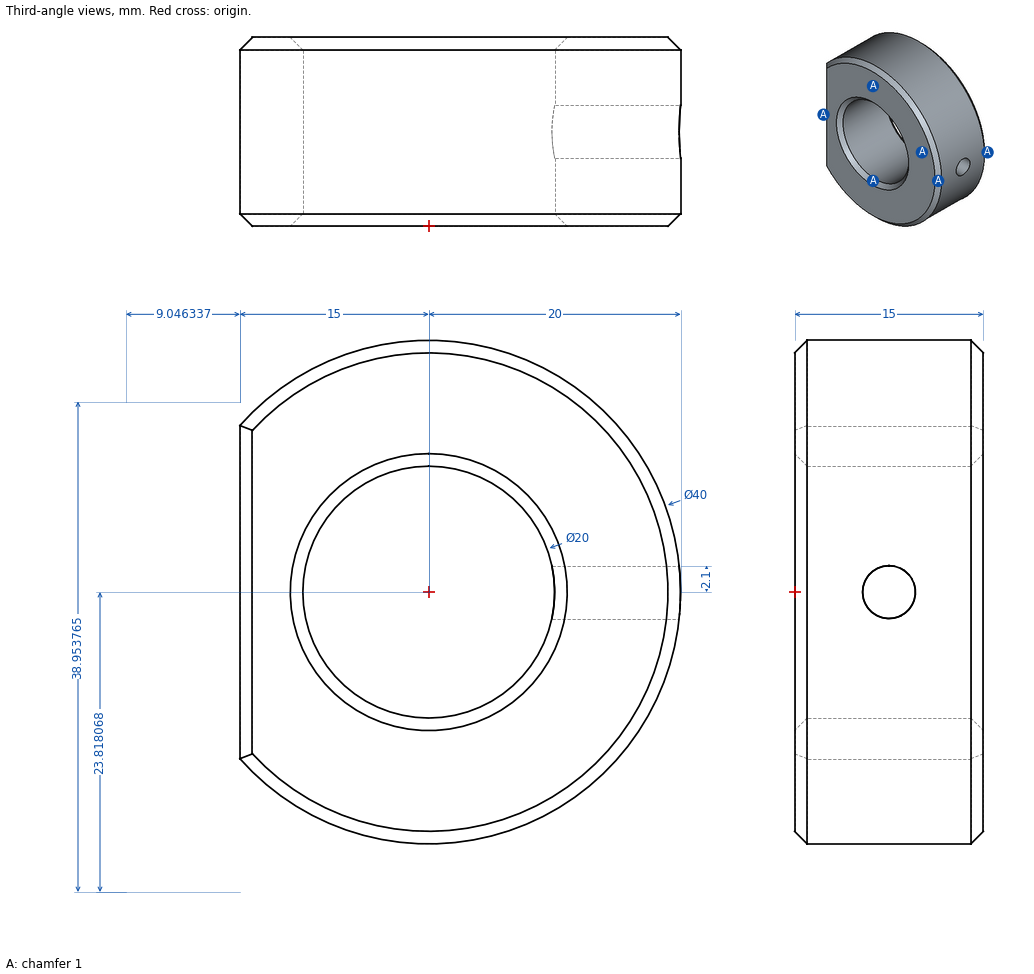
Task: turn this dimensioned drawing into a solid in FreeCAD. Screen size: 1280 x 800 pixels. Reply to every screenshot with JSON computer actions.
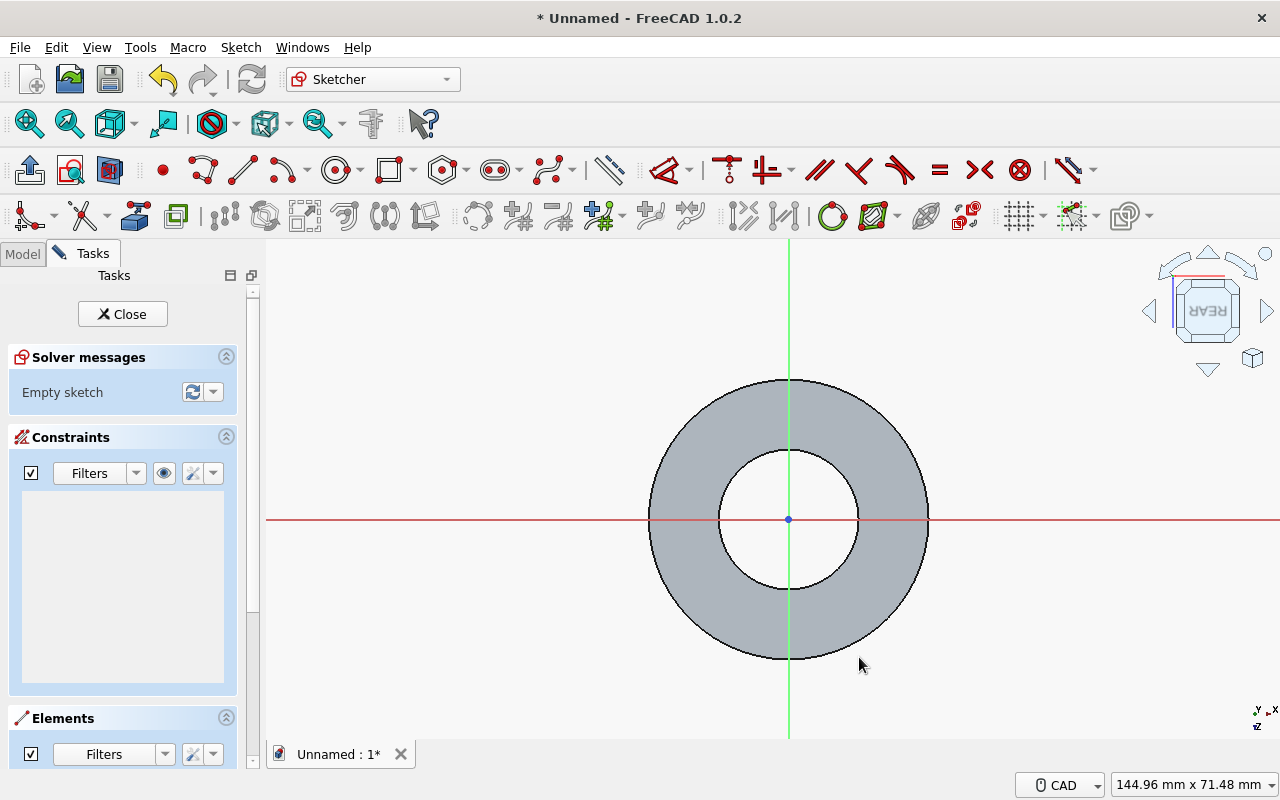
{"action": "left_click", "coordinate": [390, 170]}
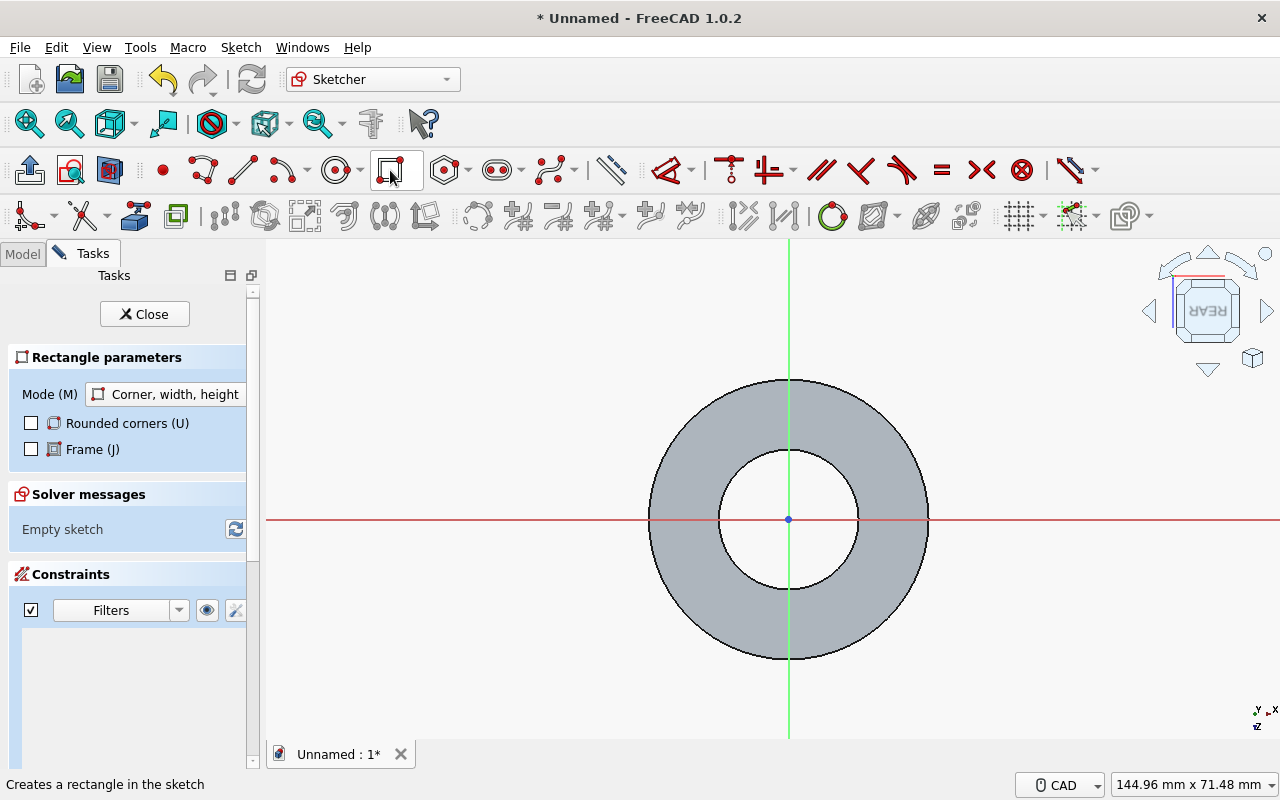
{"action": "left_click", "coordinate": [620, 353]}
{"action": "mouse_move", "coordinate": [684, 625]}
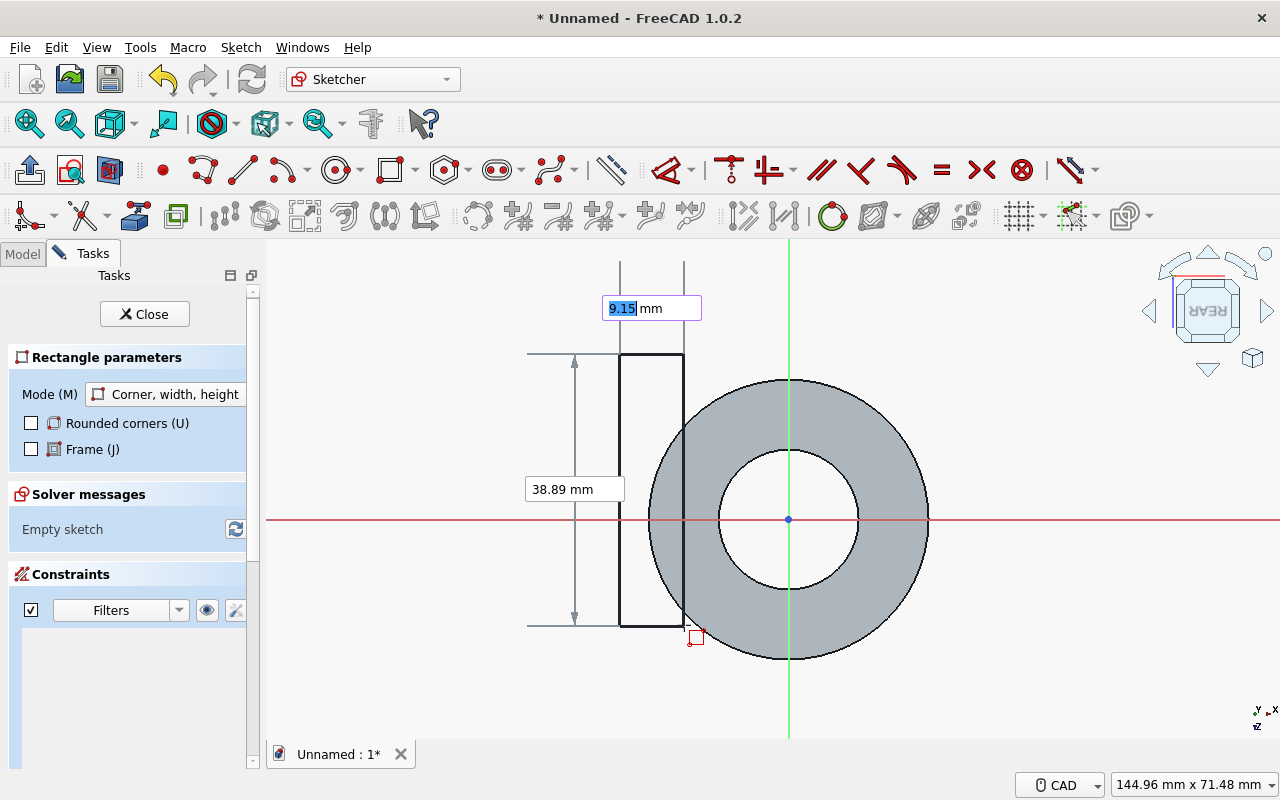
{"action": "type", "text": "9.046337"}
{"action": "key", "text": "Tab"}
{"action": "type", "text": "38.953765"}
{"action": "key", "text": "Return"}
{"action": "key", "text": "Escape"}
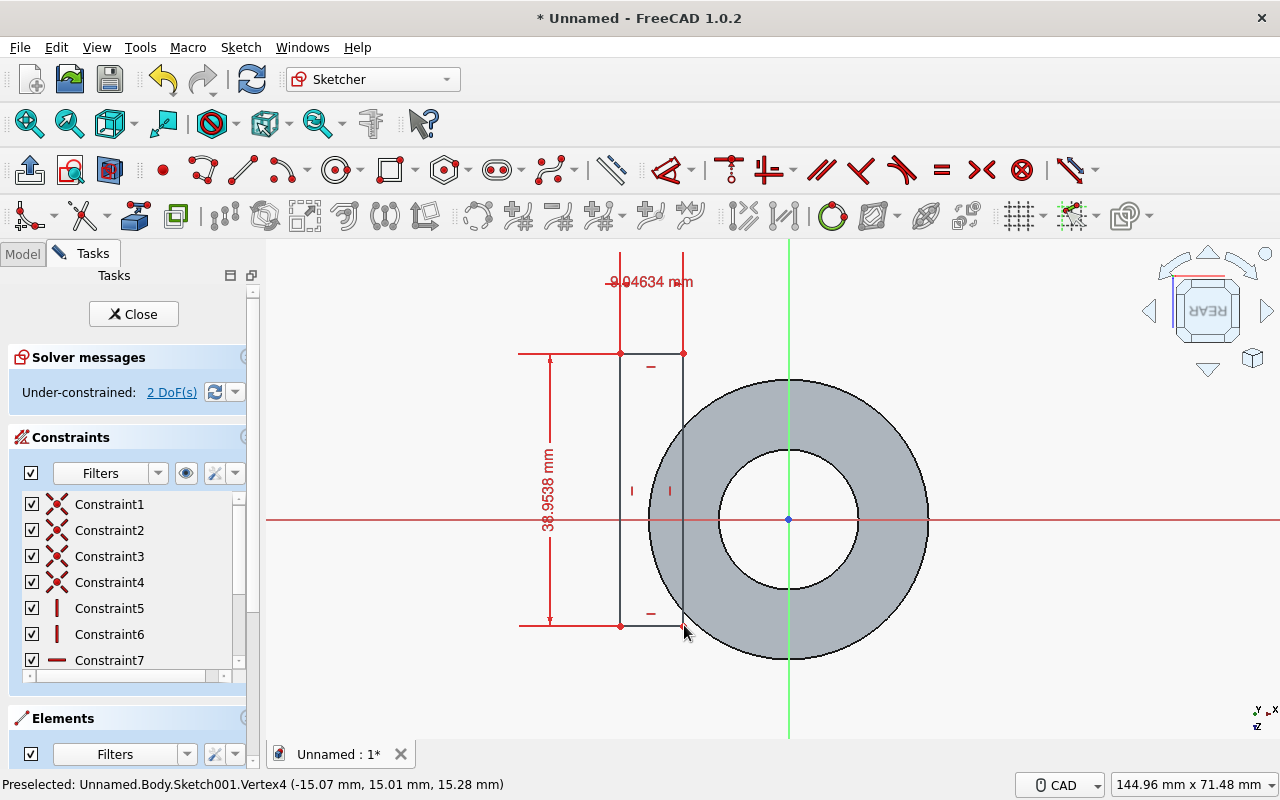
{"action": "left_click", "coordinate": [666, 170]}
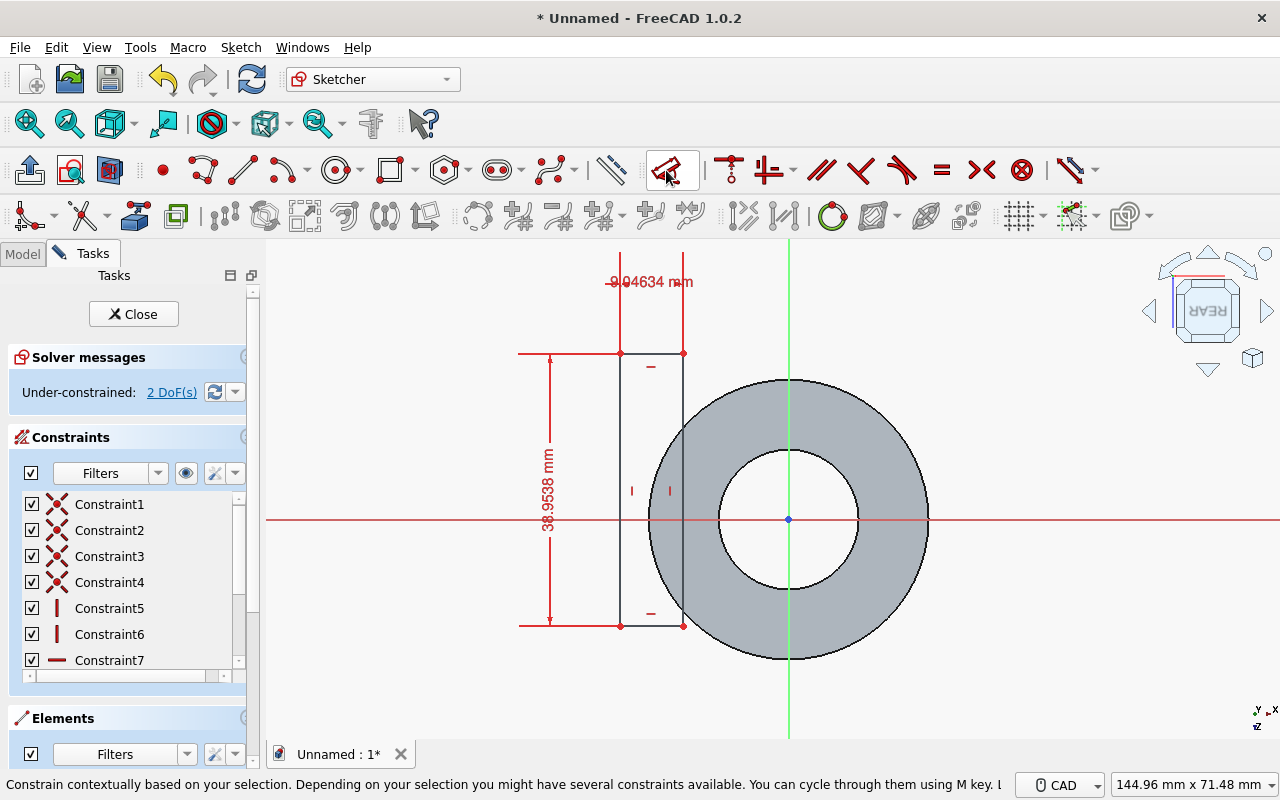
{"action": "left_click", "coordinate": [683, 626]}
{"action": "left_click", "coordinate": [736, 660]}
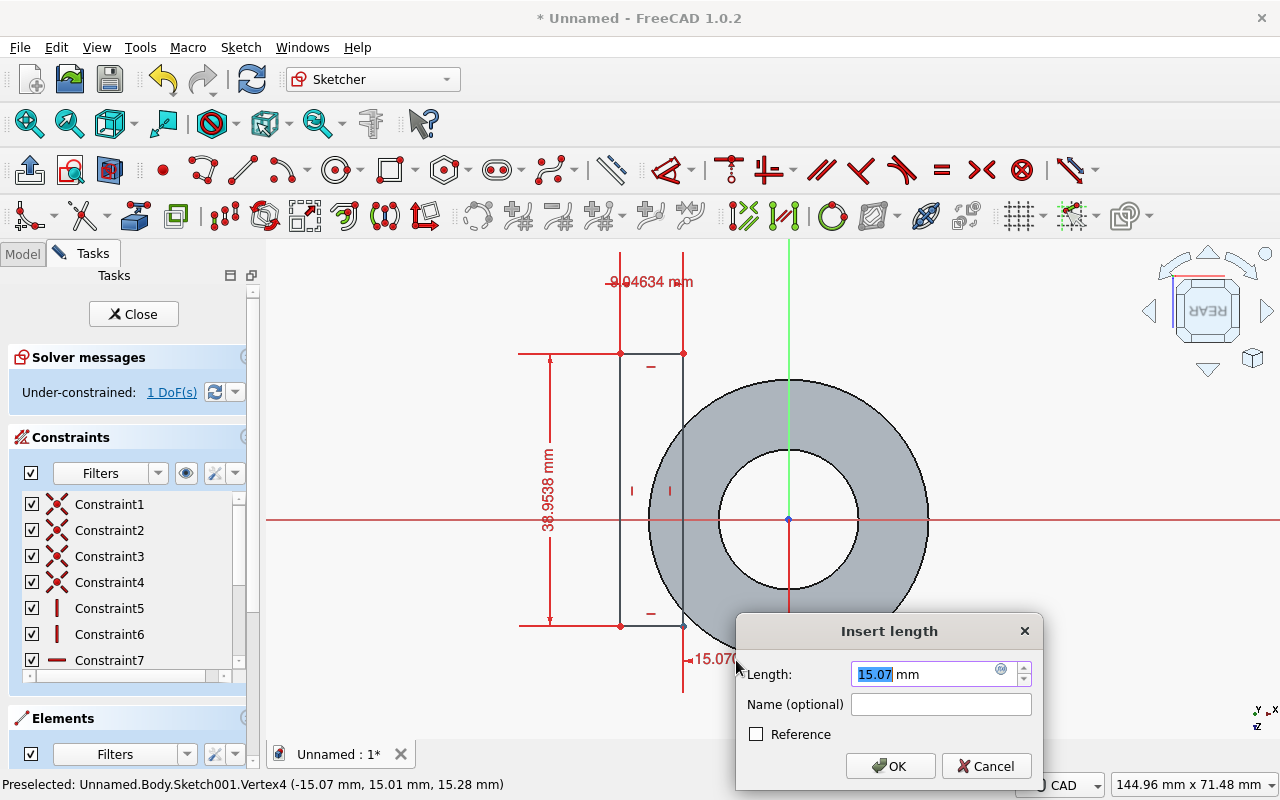
{"action": "type", "text": "15"}
{"action": "key", "text": "Return"}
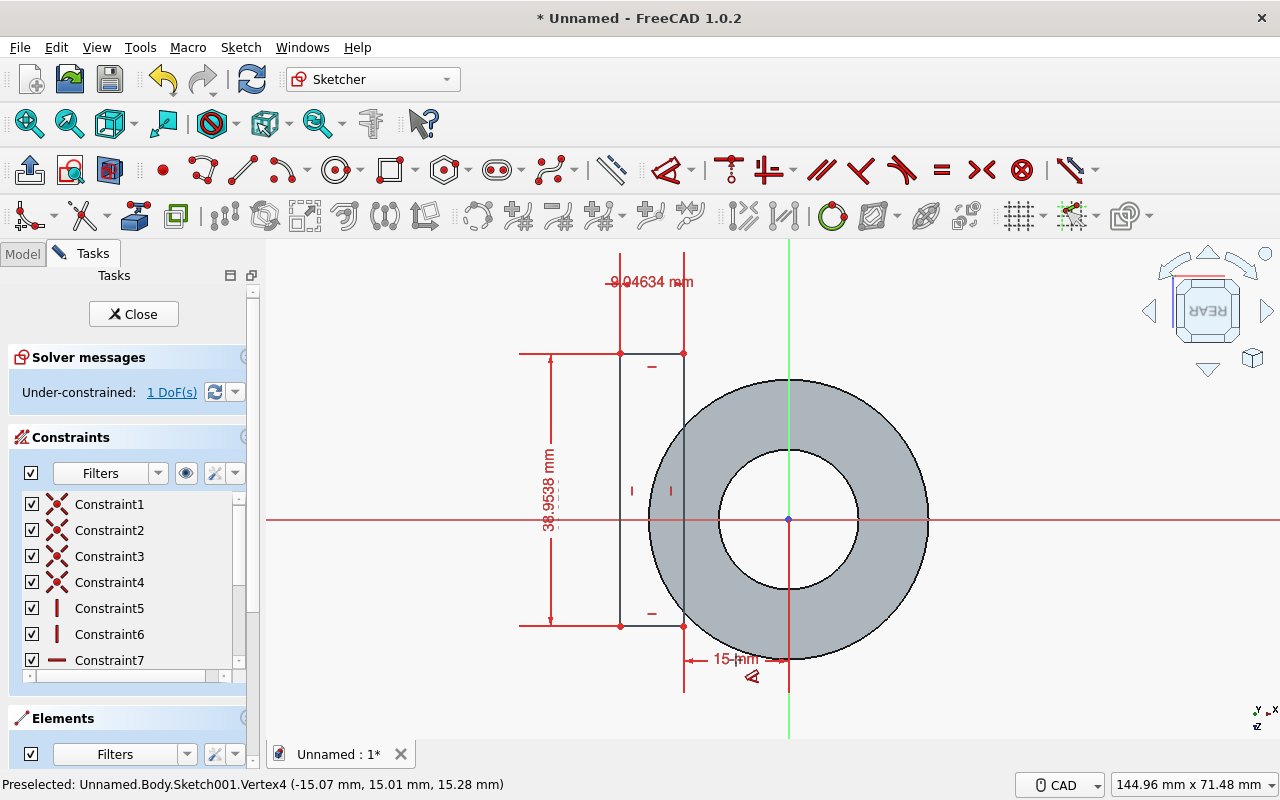
{"action": "left_click", "coordinate": [620, 354]}
{"action": "left_click", "coordinate": [586, 437]}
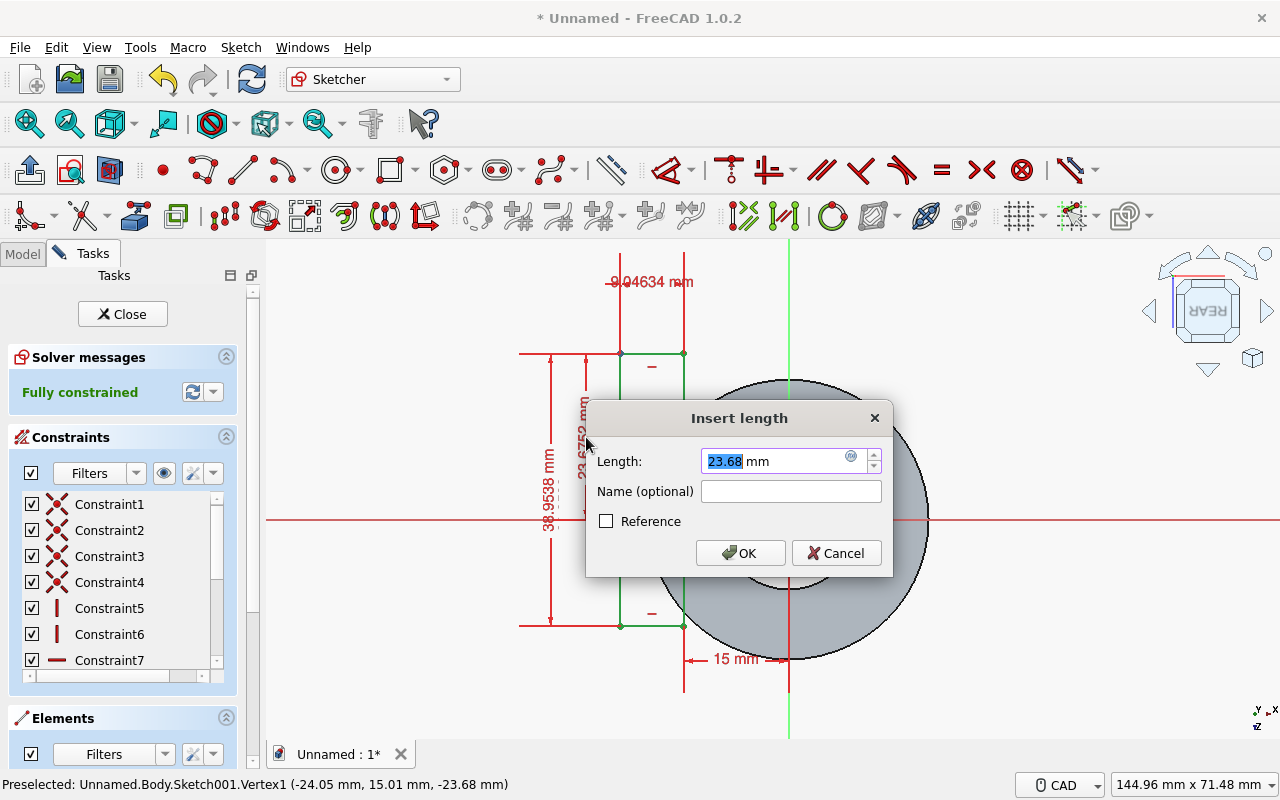
{"action": "type", "text": "23.818068"}
{"action": "key", "text": "Return"}
{"action": "key", "text": "Escape"}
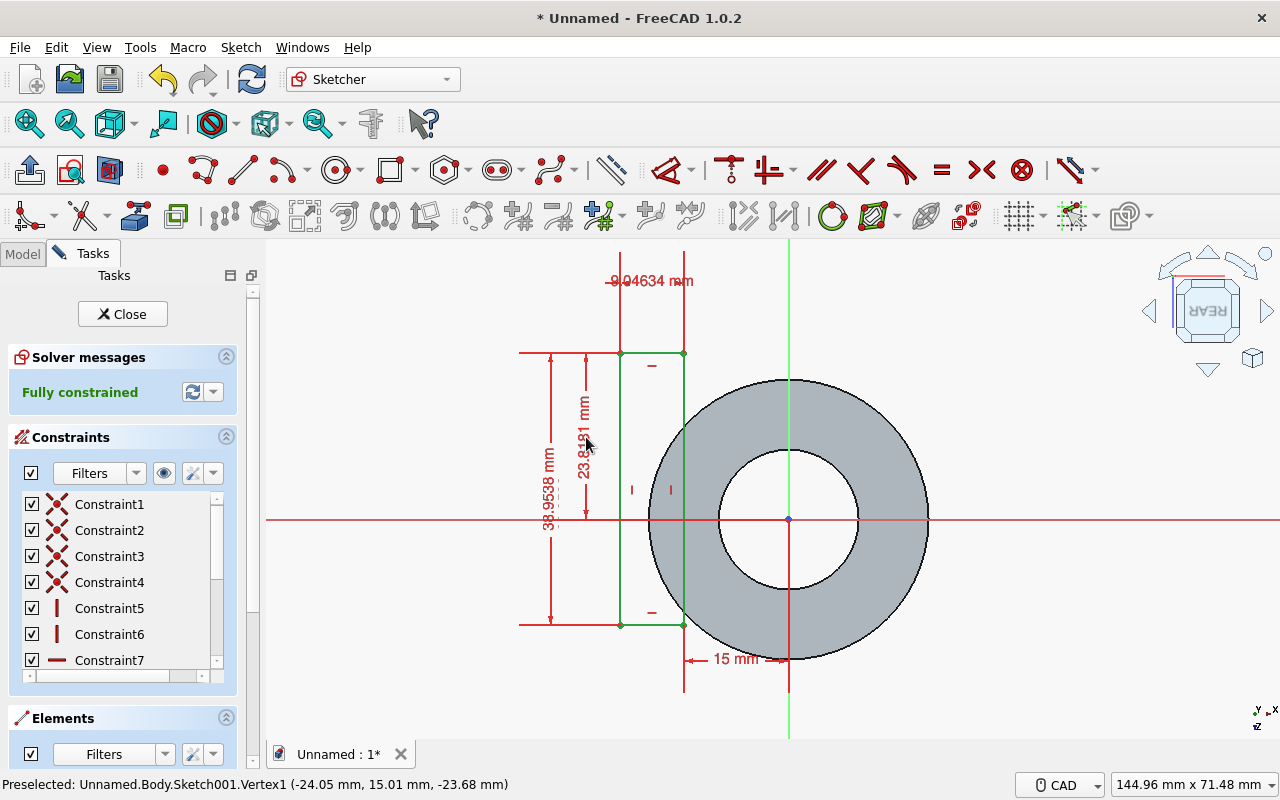
{"action": "left_click", "coordinate": [123, 314]}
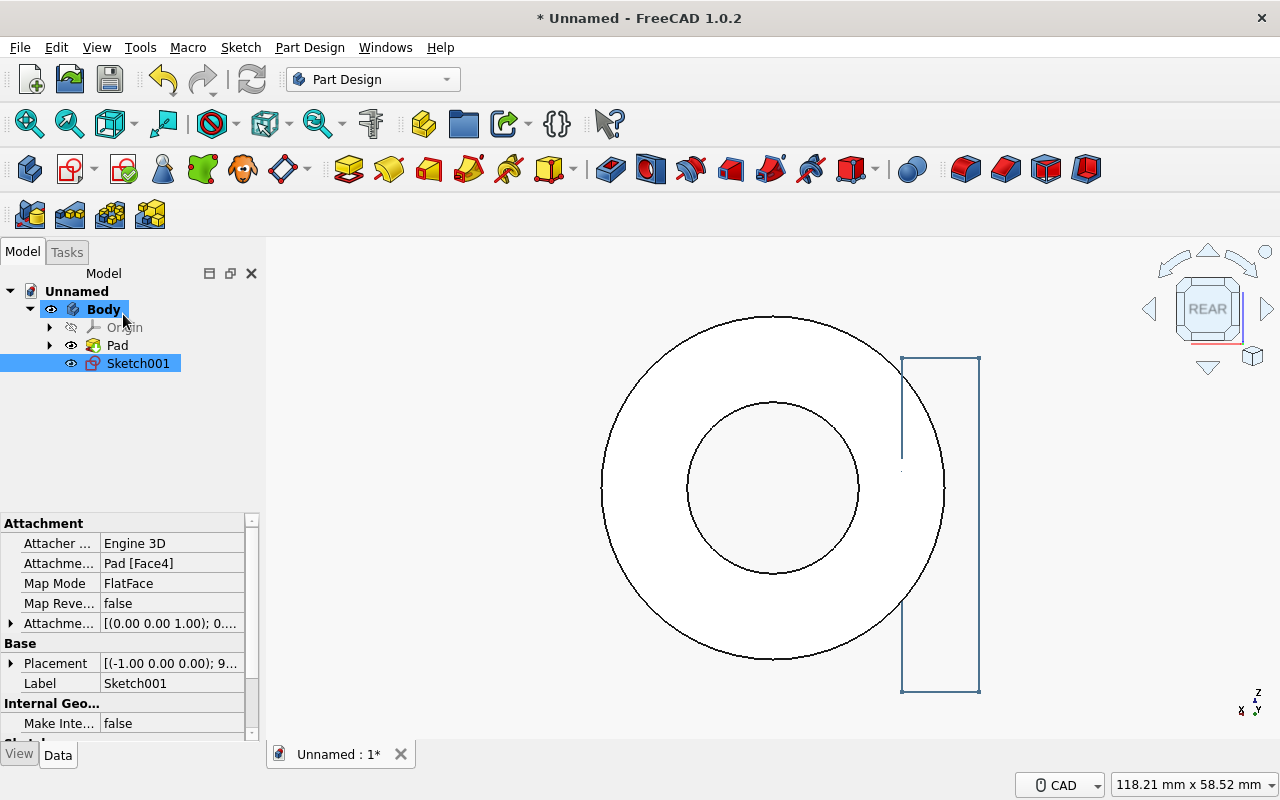
{"action": "left_click", "coordinate": [612, 170]}